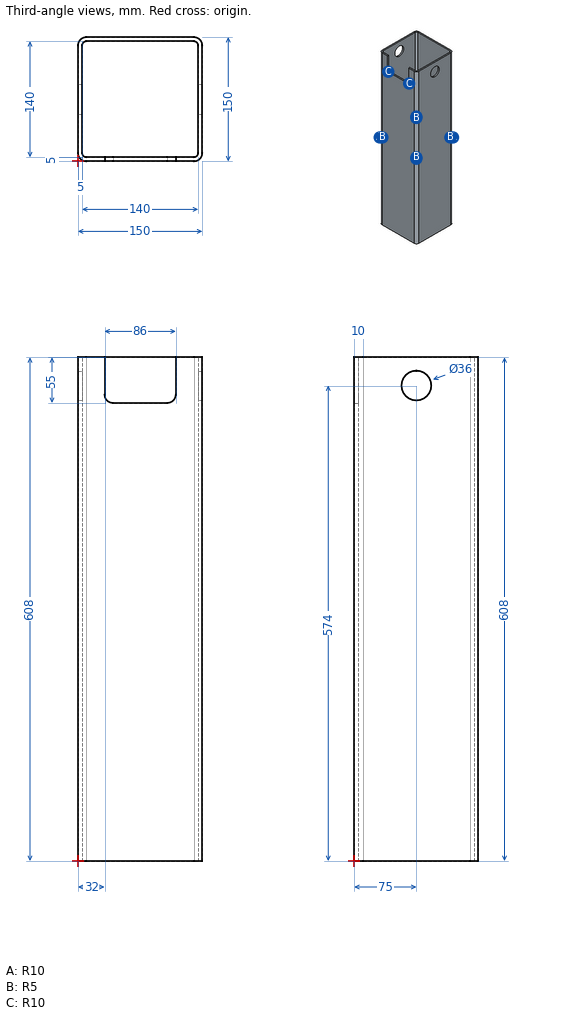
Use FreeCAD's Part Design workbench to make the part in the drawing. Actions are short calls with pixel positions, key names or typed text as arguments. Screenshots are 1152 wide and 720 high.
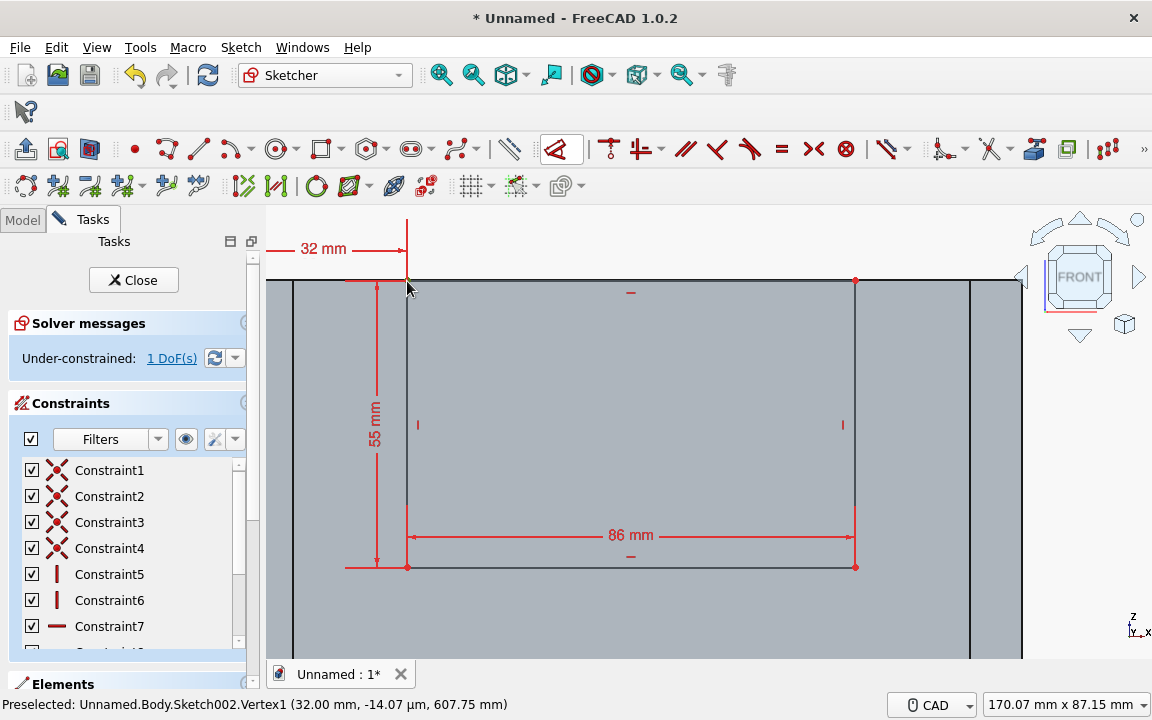
key(i)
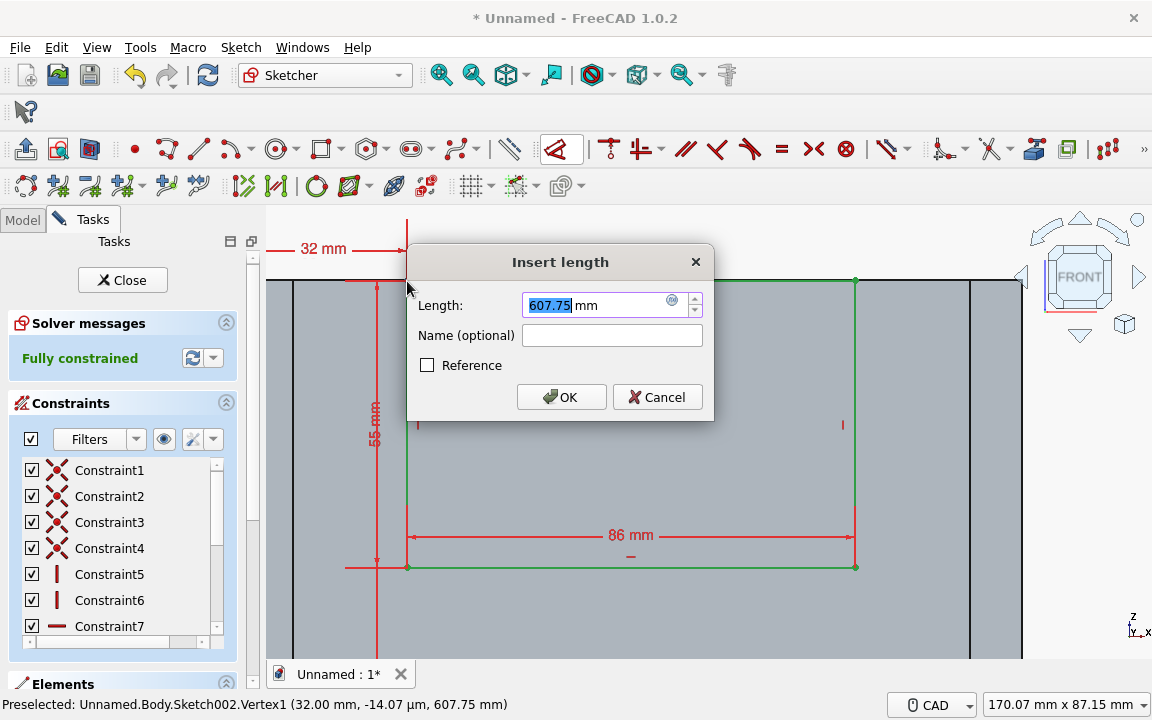
text(608)
key(Return)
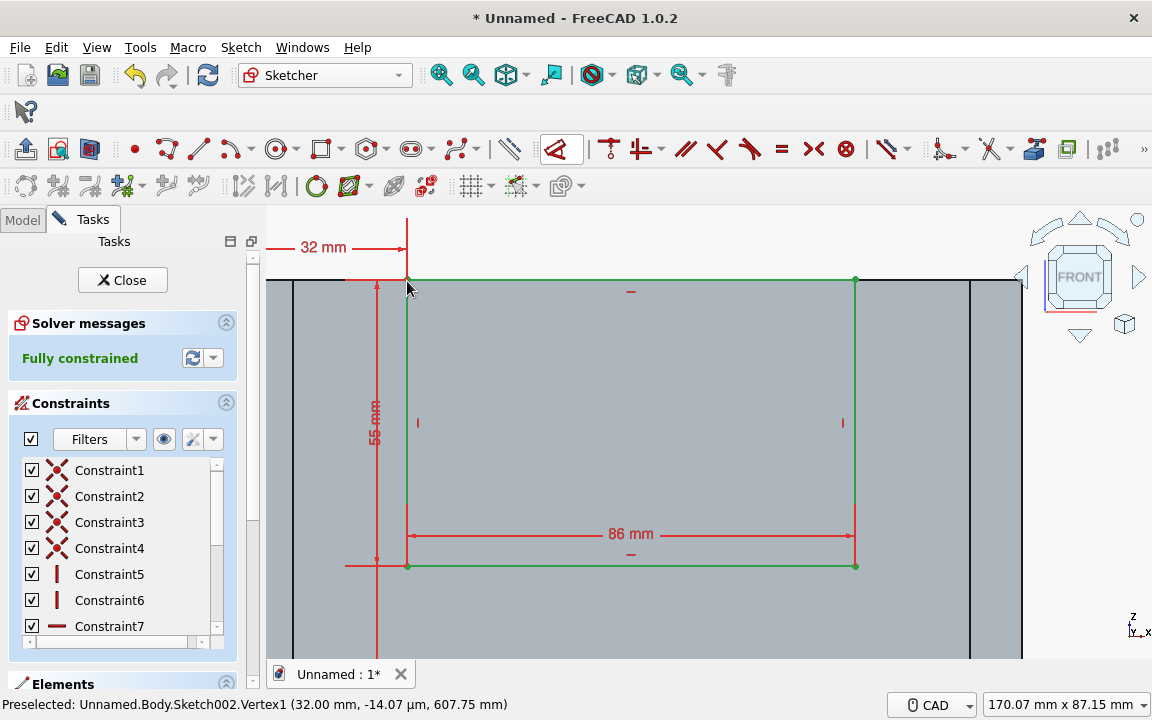
click(123, 280)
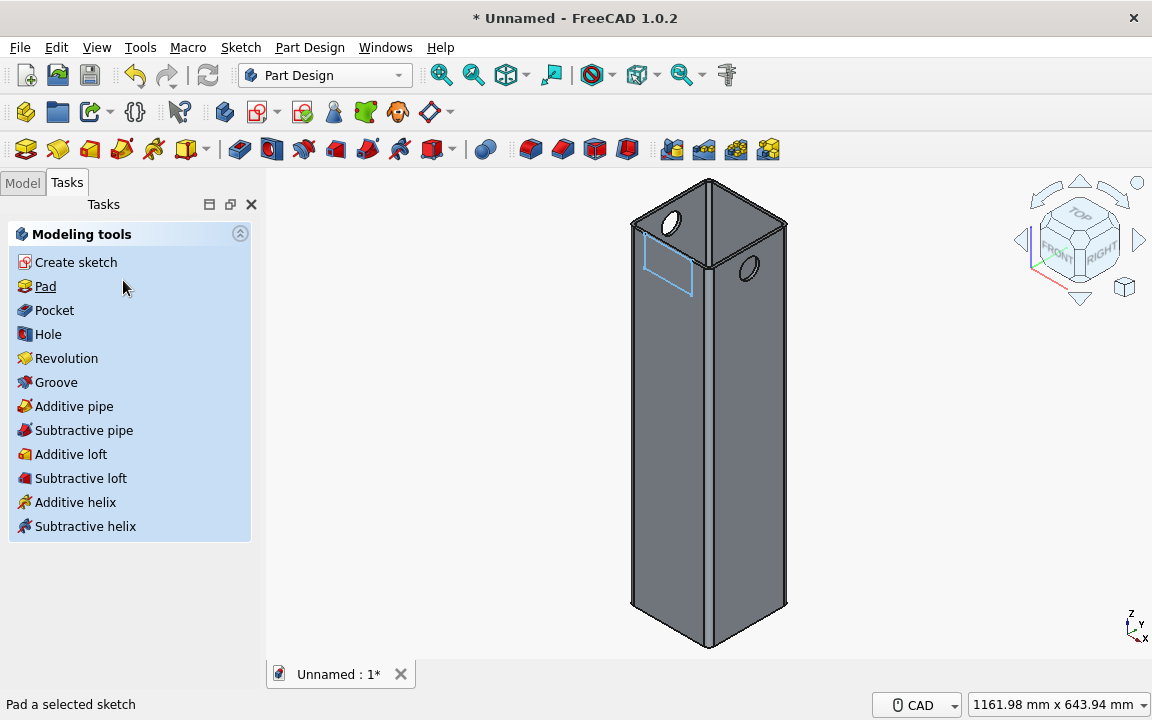
click(240, 150)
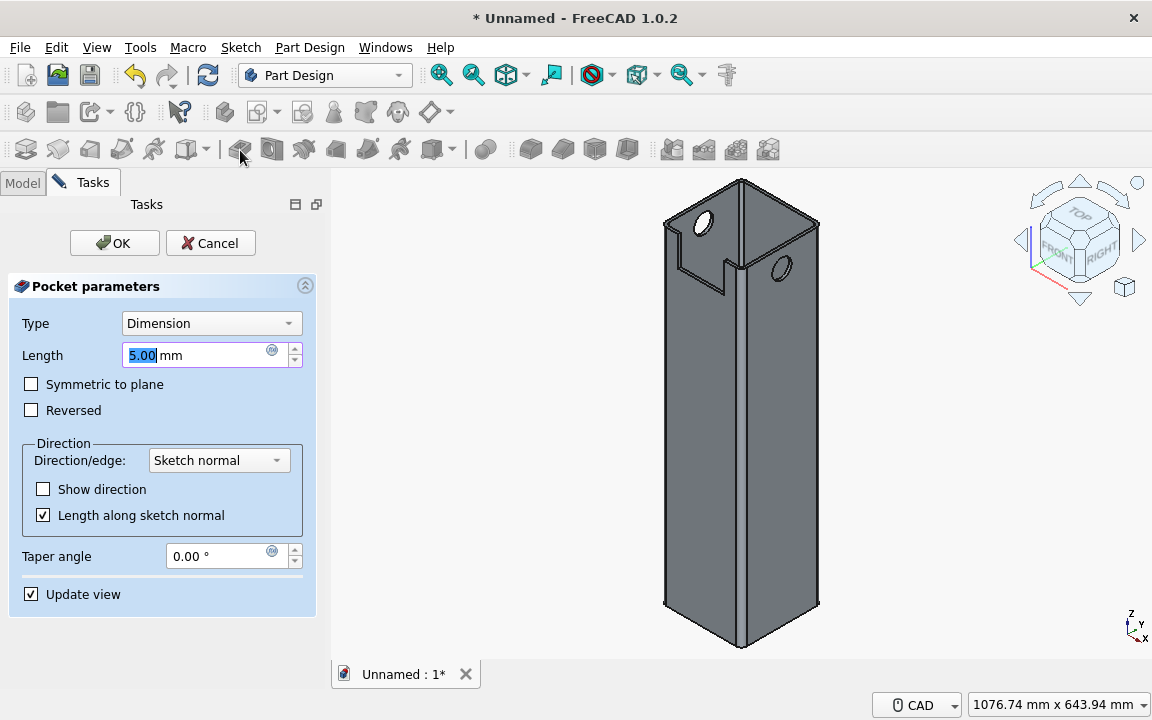
text(10)
key(Tab)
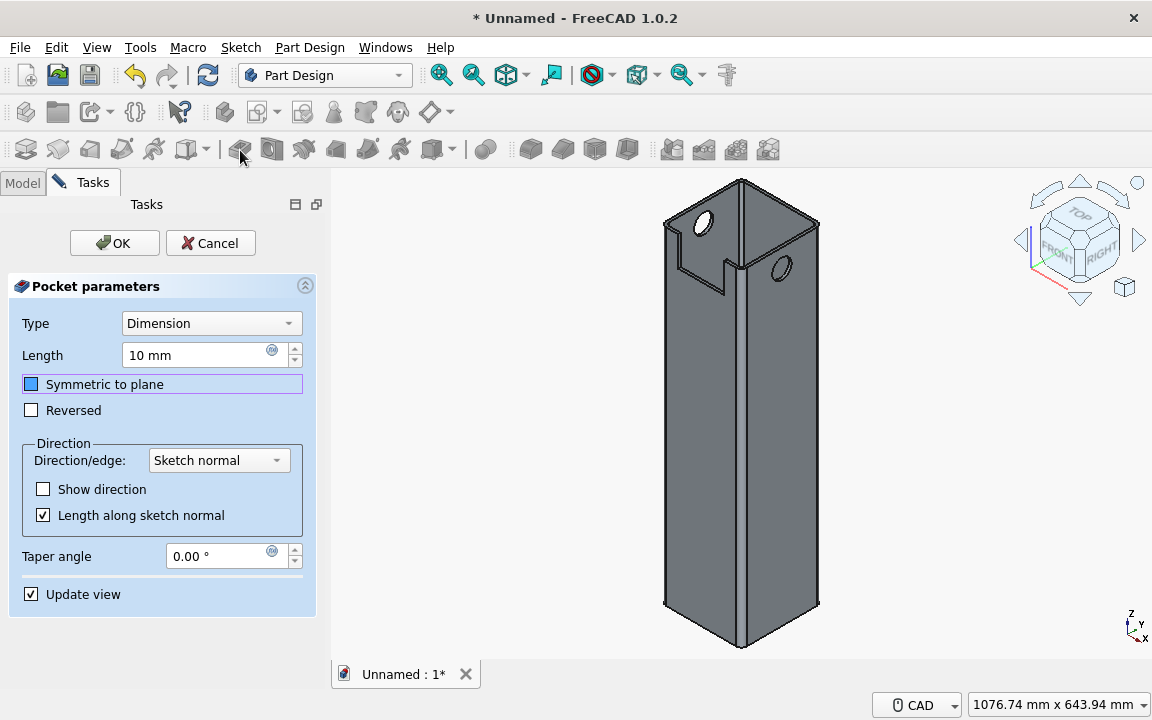
click(115, 243)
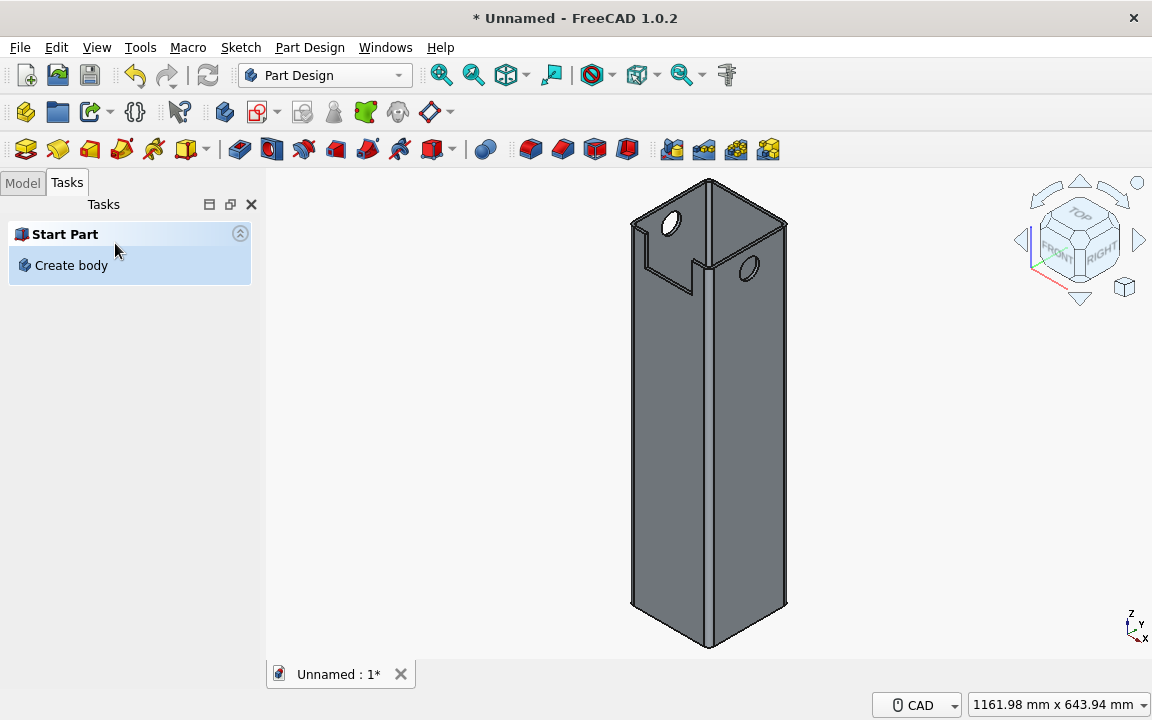
scroll(647, 267, up, 12)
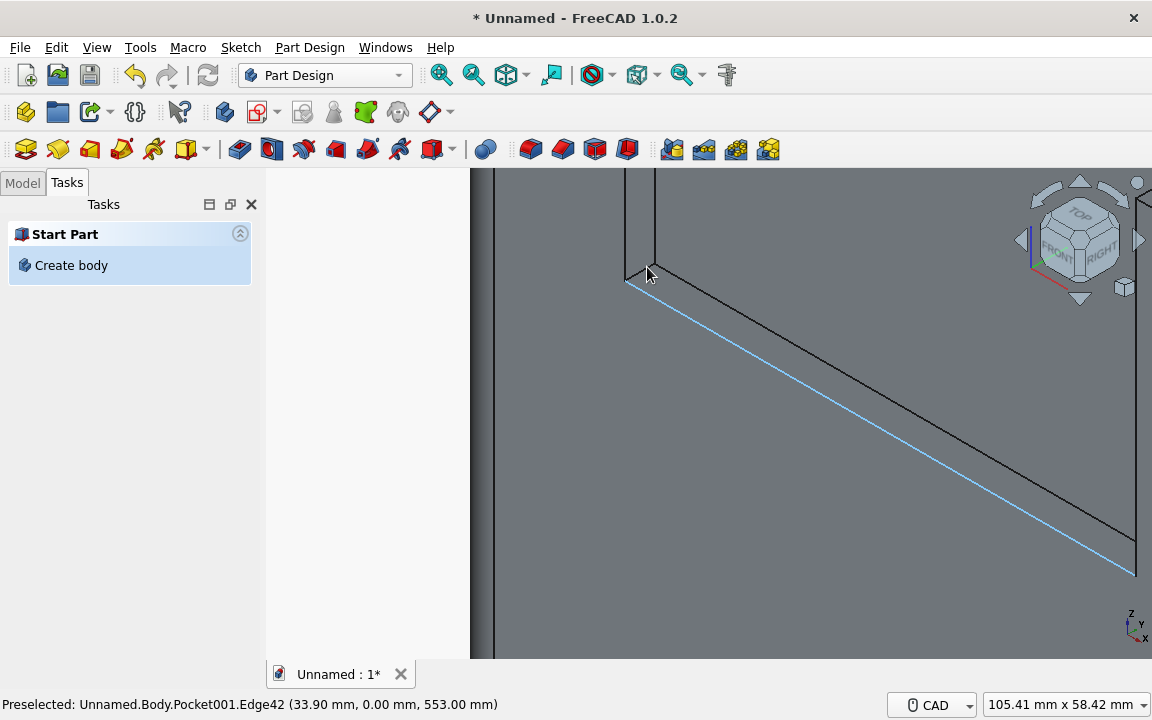
key(v)
key(f)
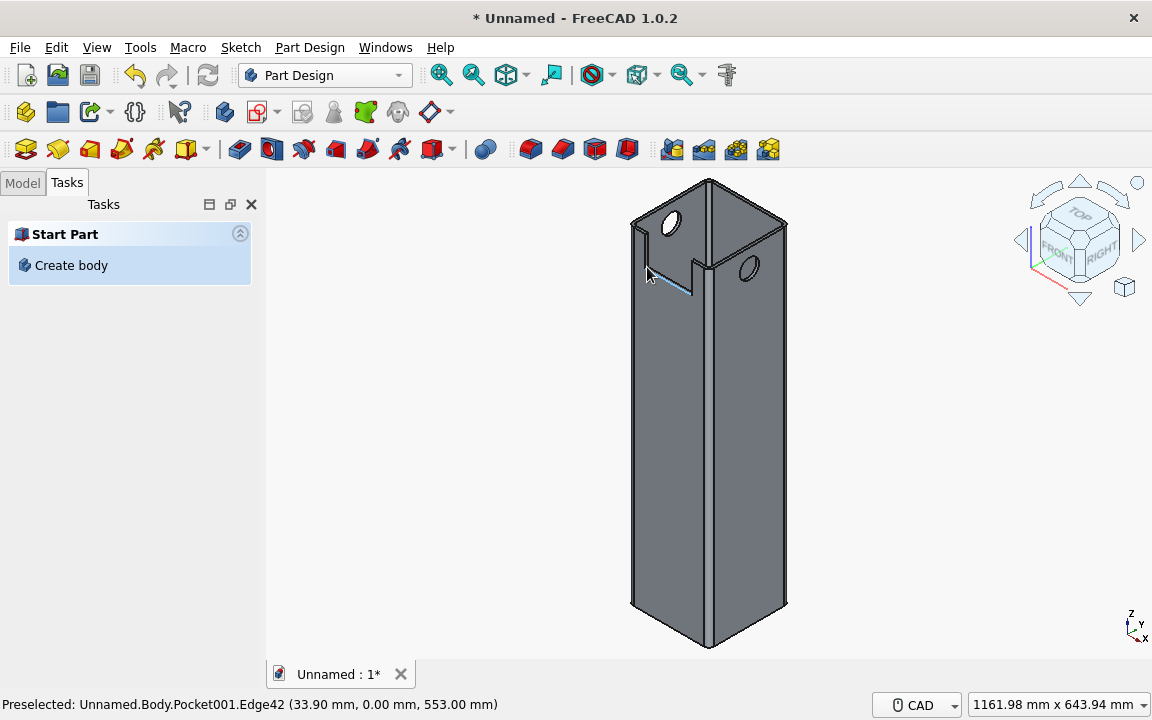
key(2)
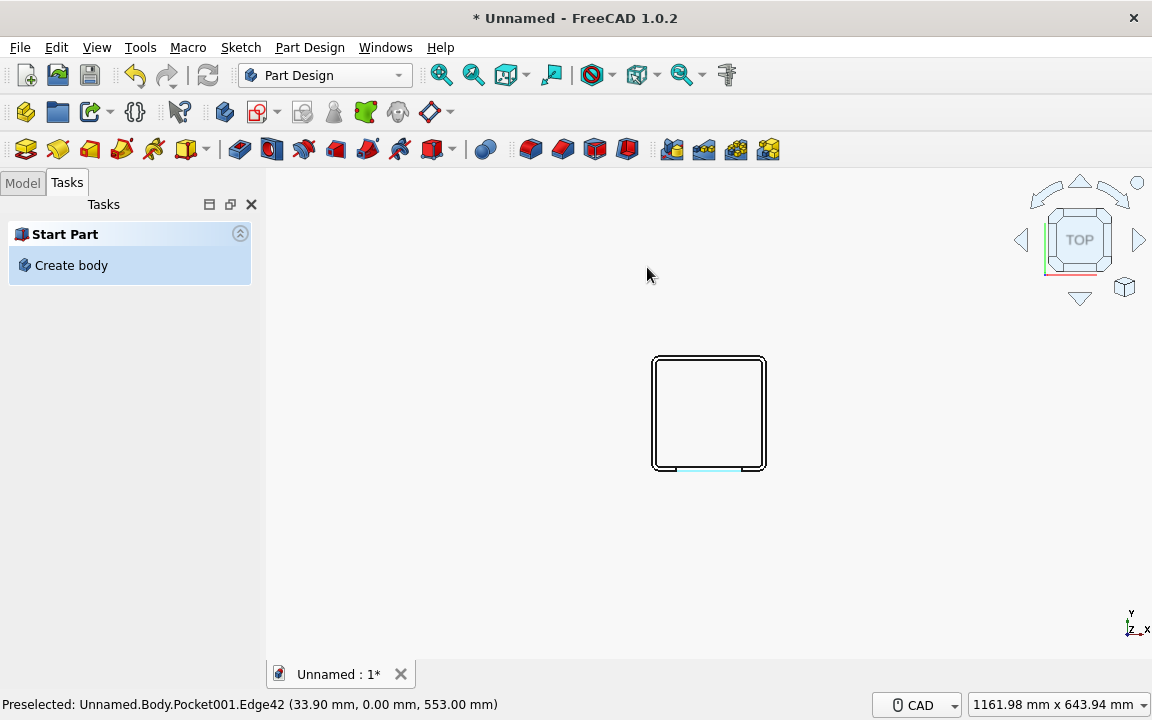
click(442, 76)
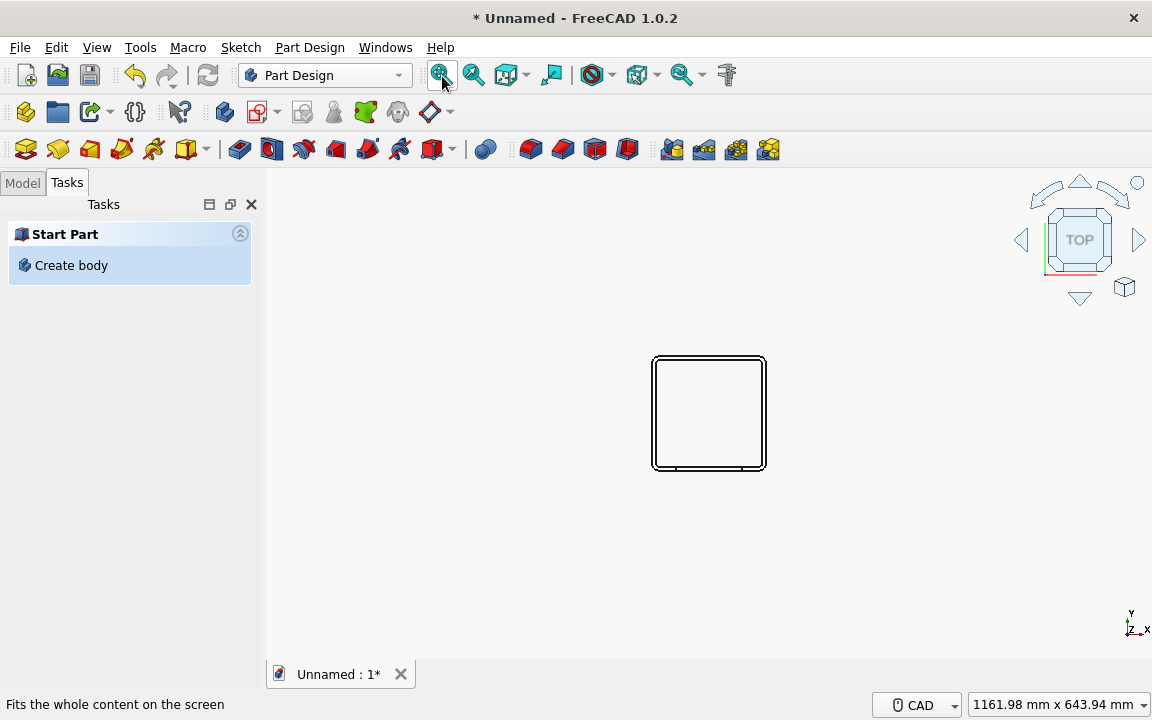
scroll(676, 468, up, 12)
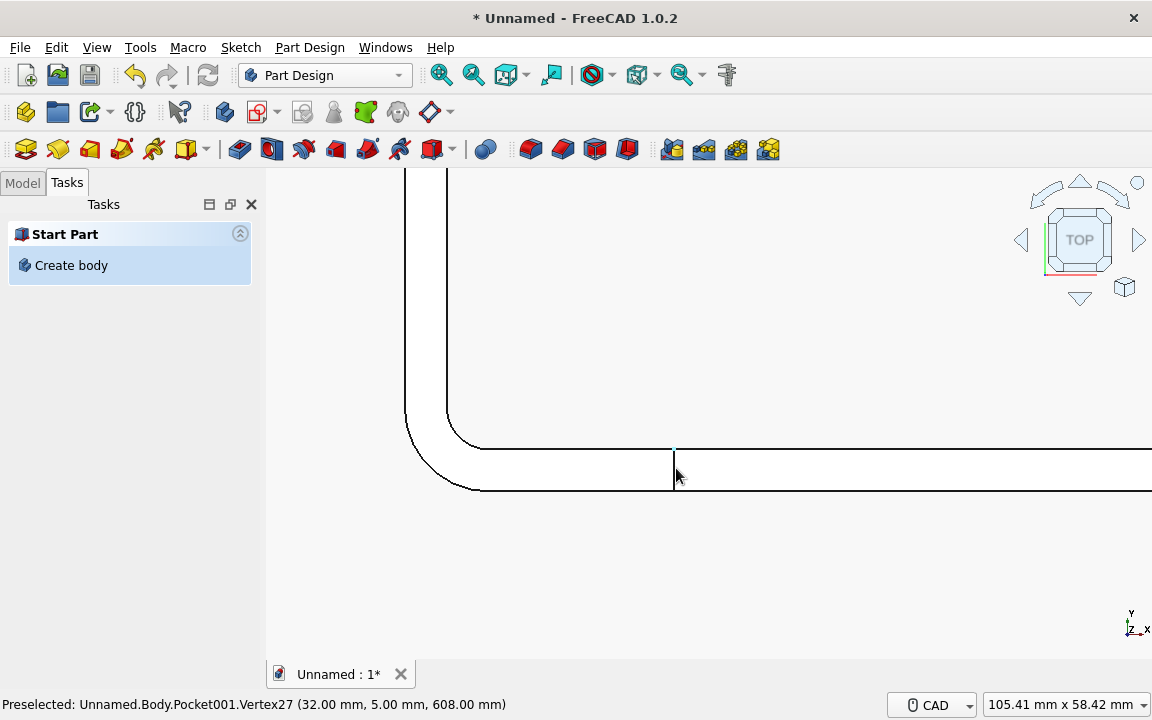
click(442, 76)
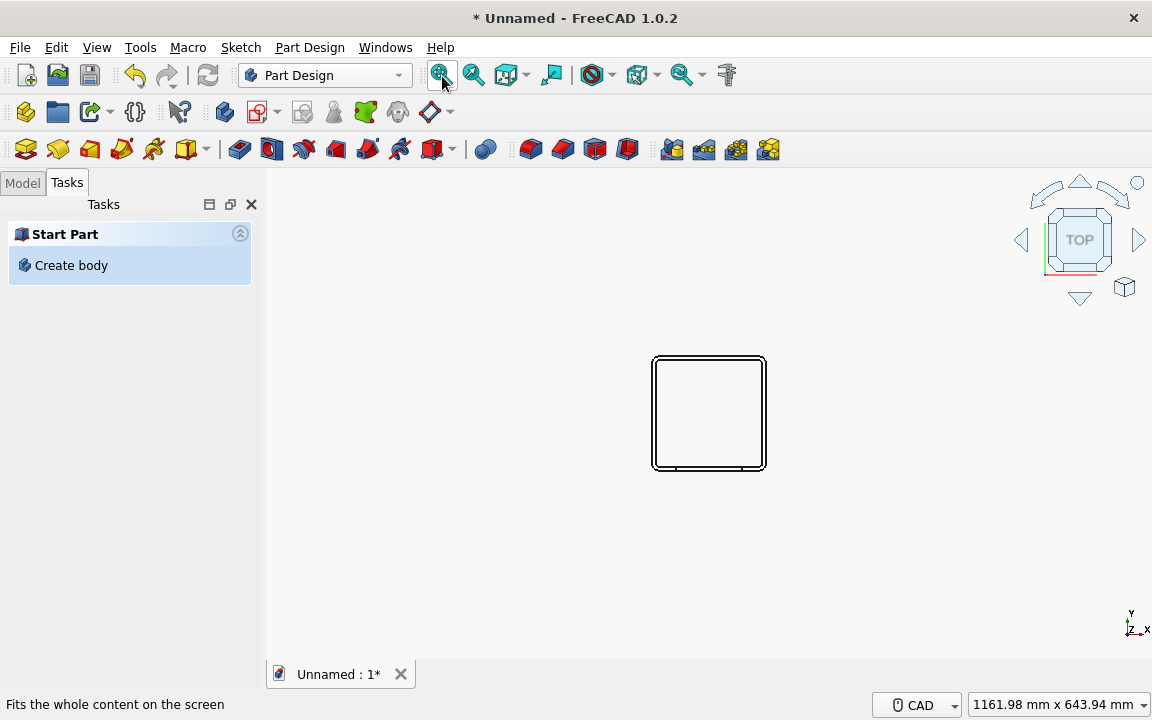
key(0)